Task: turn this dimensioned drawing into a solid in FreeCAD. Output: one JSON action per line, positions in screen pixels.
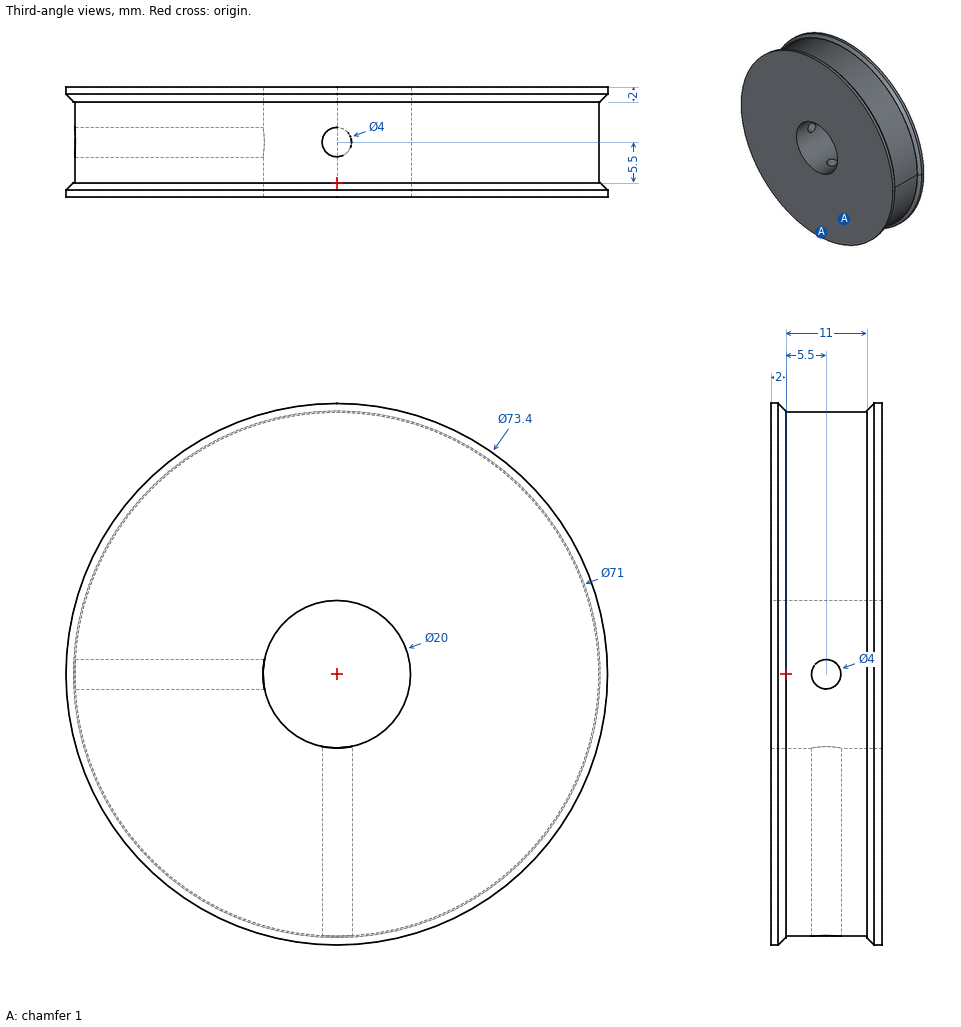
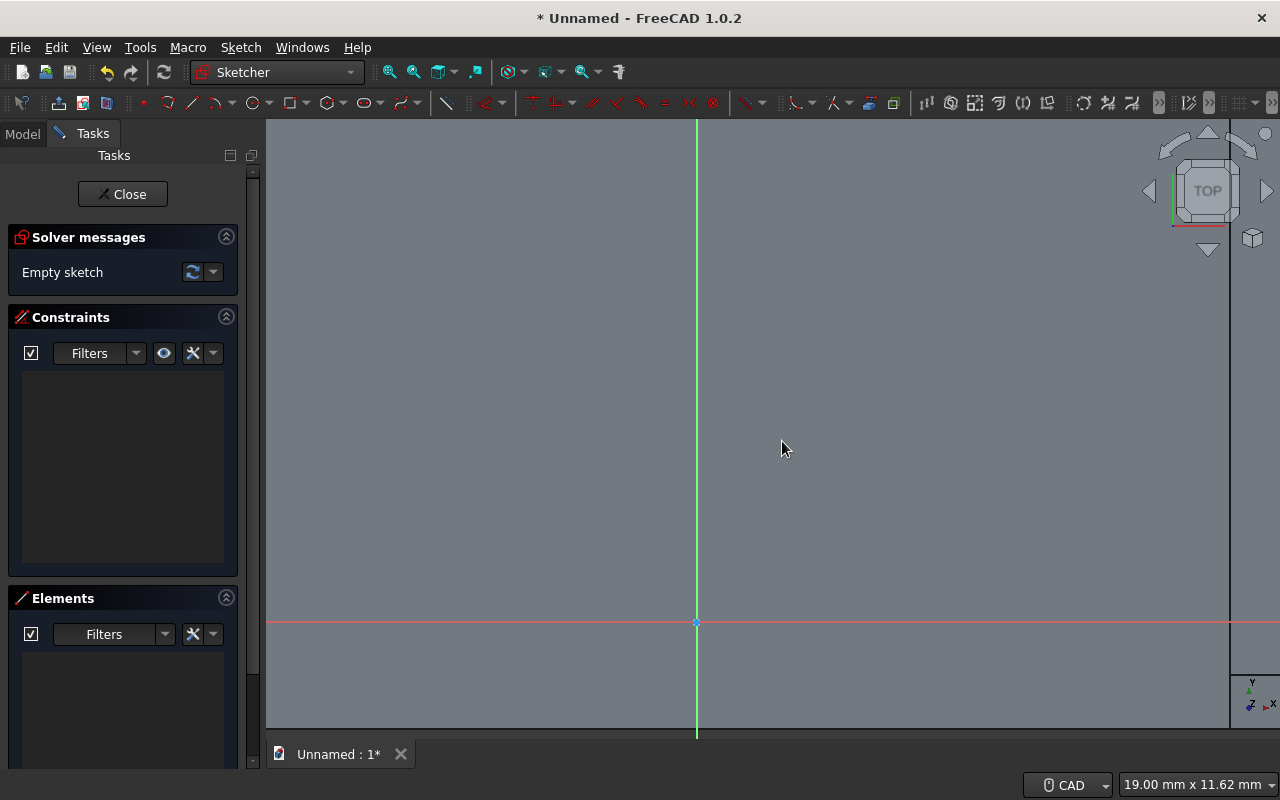
{"action": "left_click", "coordinate": [254, 104]}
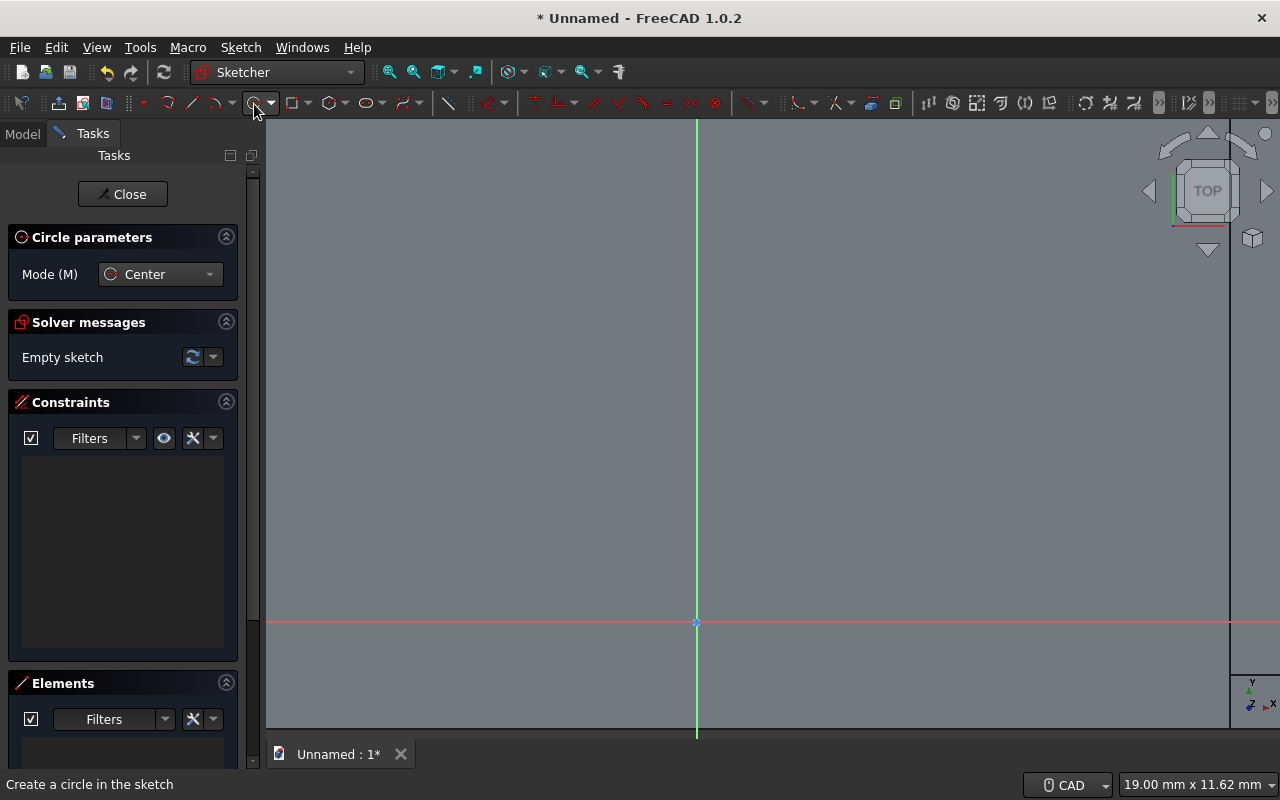
{"action": "left_click", "coordinate": [697, 329]}
{"action": "left_click", "coordinate": [772, 253]}
{"action": "key", "text": "Escape"}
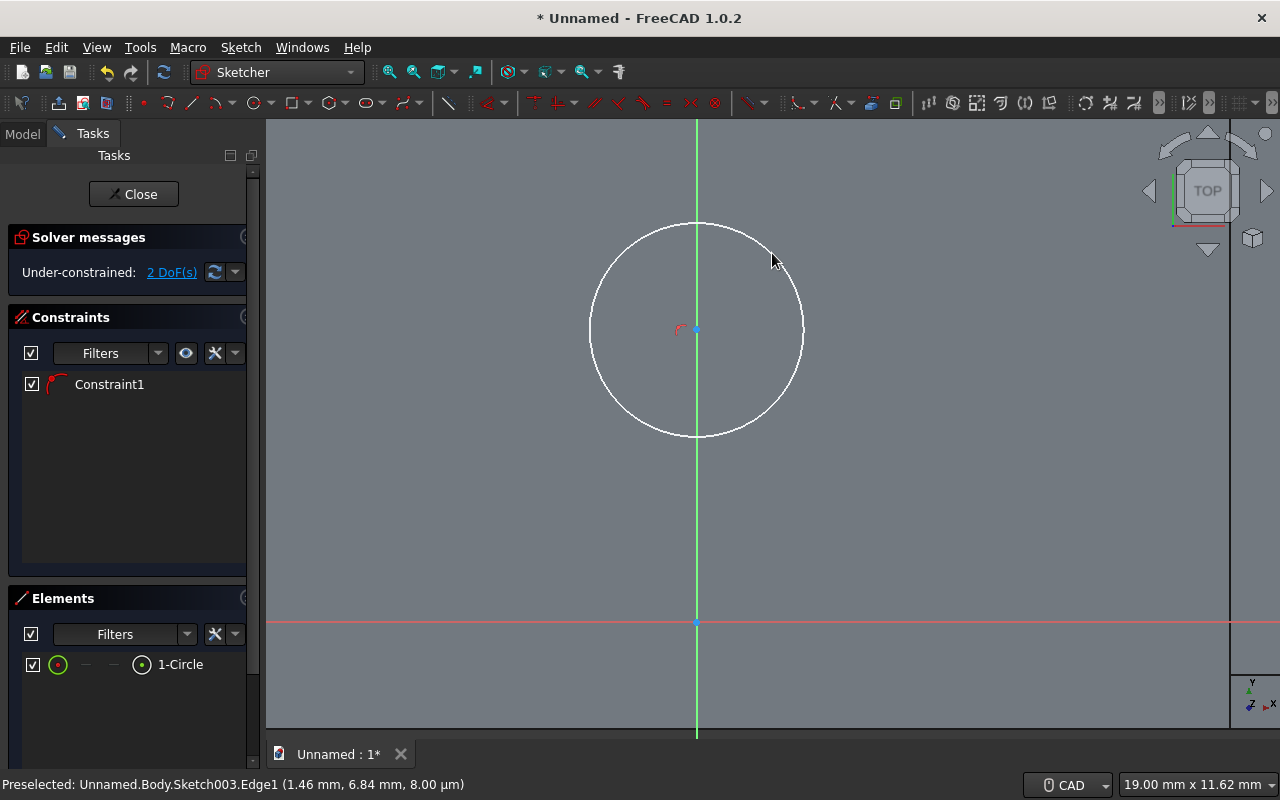
{"action": "left_click", "coordinate": [488, 104]}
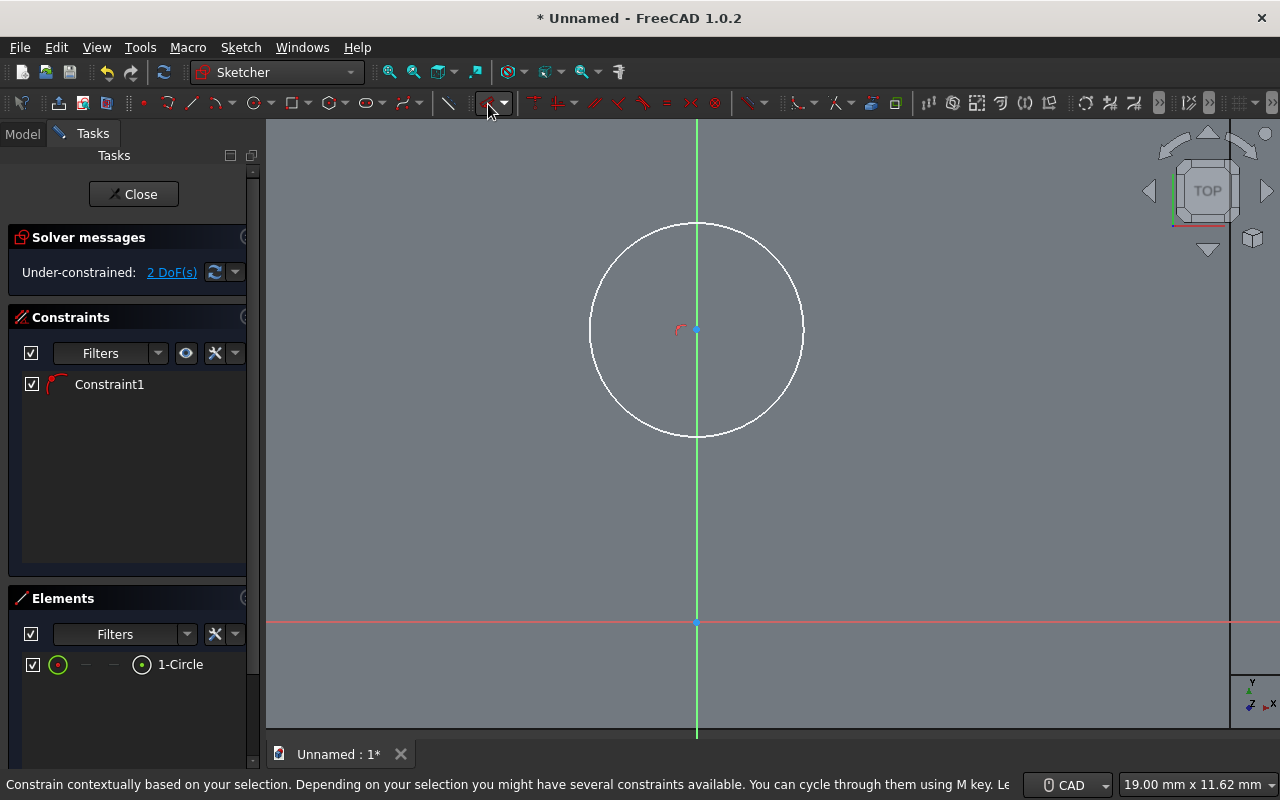
{"action": "left_click", "coordinate": [772, 254]}
{"action": "left_click", "coordinate": [795, 231]}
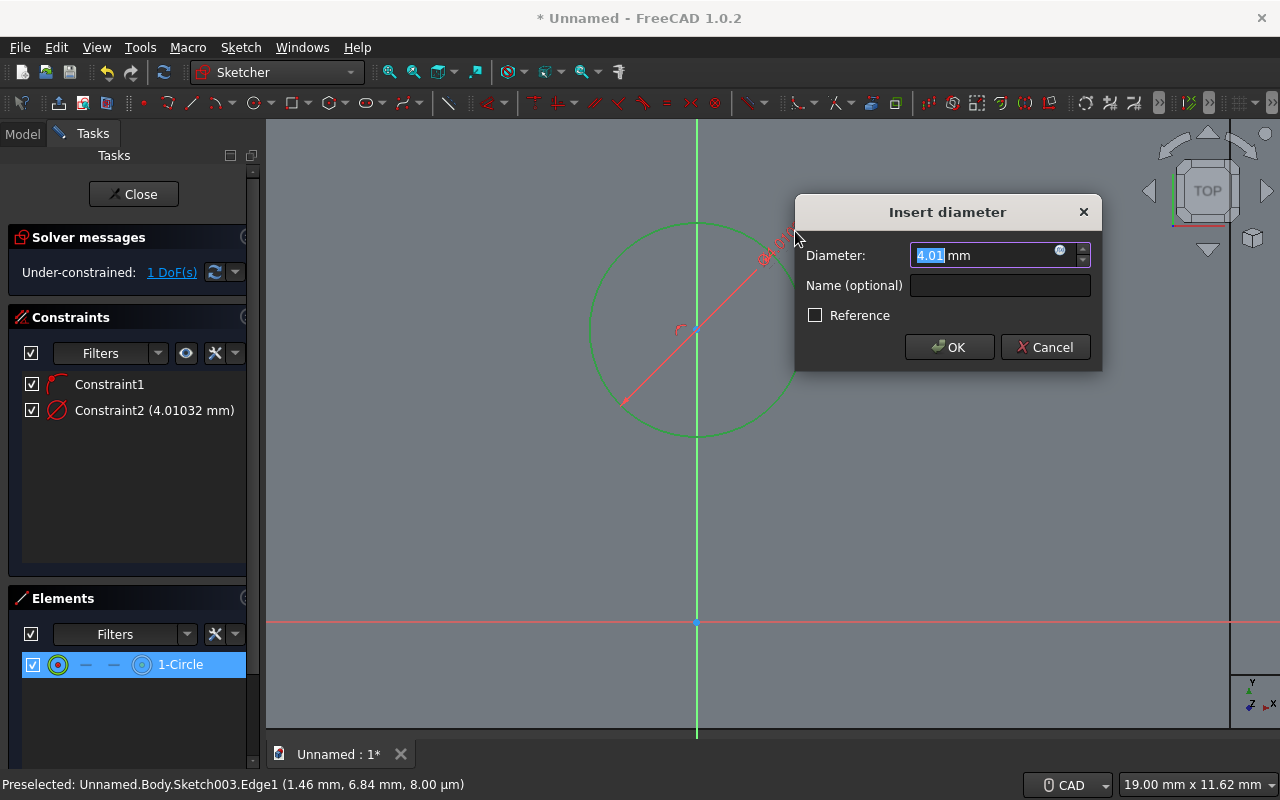
{"action": "type", "text": "4"}
{"action": "key", "text": "Return"}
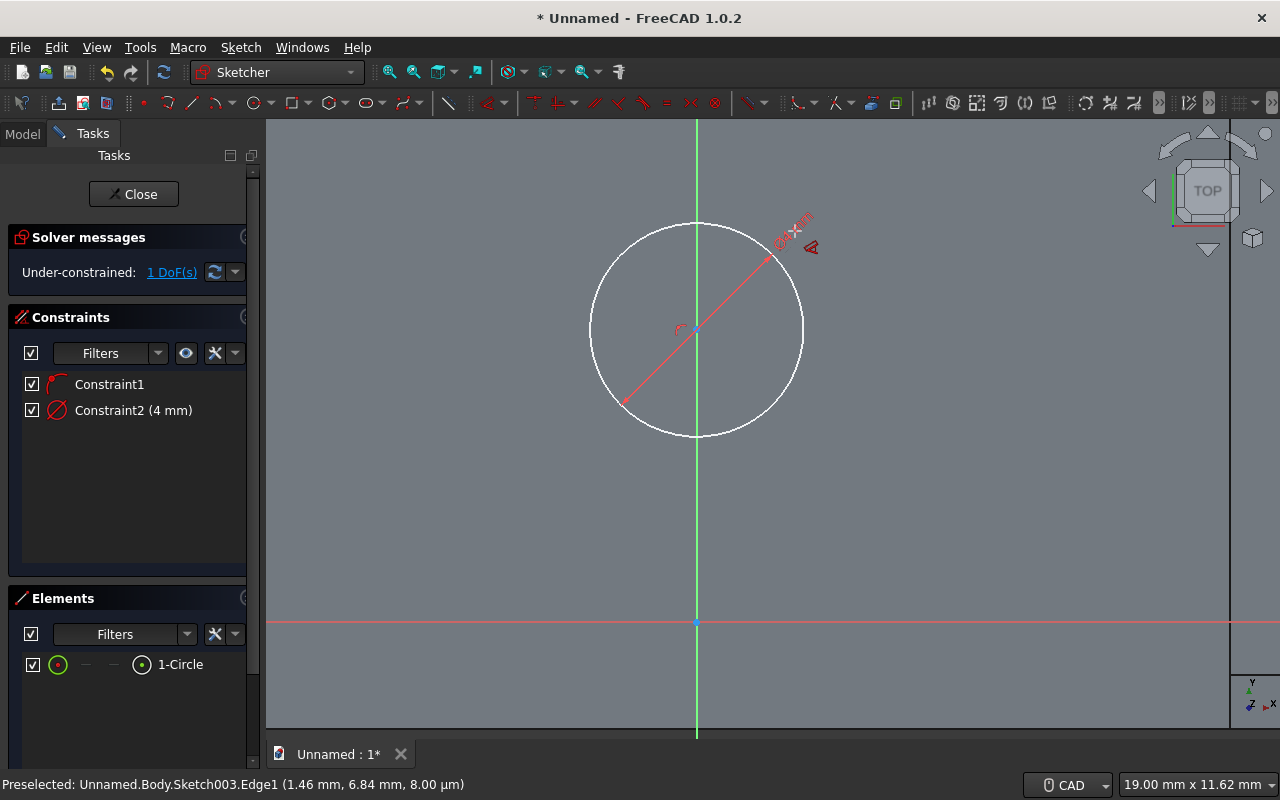
{"action": "left_click", "coordinate": [697, 330]}
{"action": "left_click", "coordinate": [731, 476]}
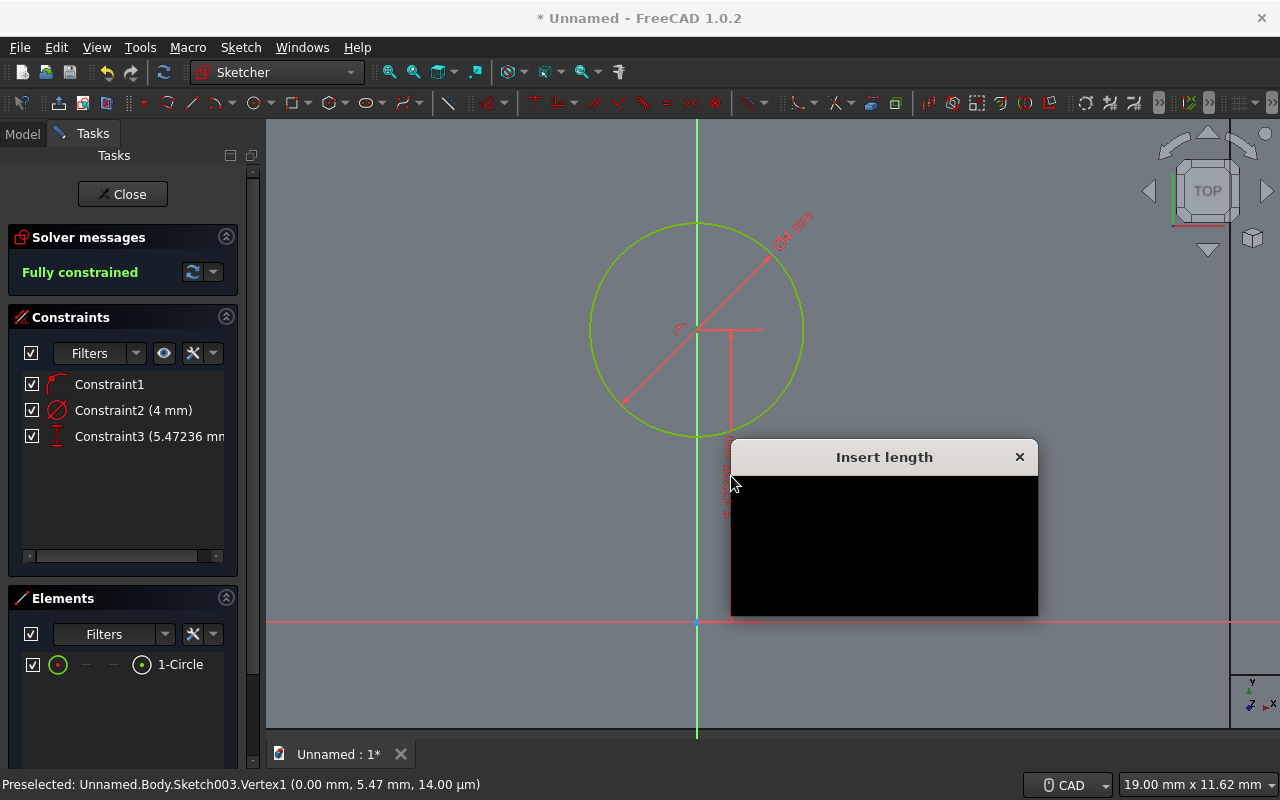
{"action": "type", "text": "5.5"}
{"action": "key", "text": "Return"}
{"action": "key", "text": "Escape"}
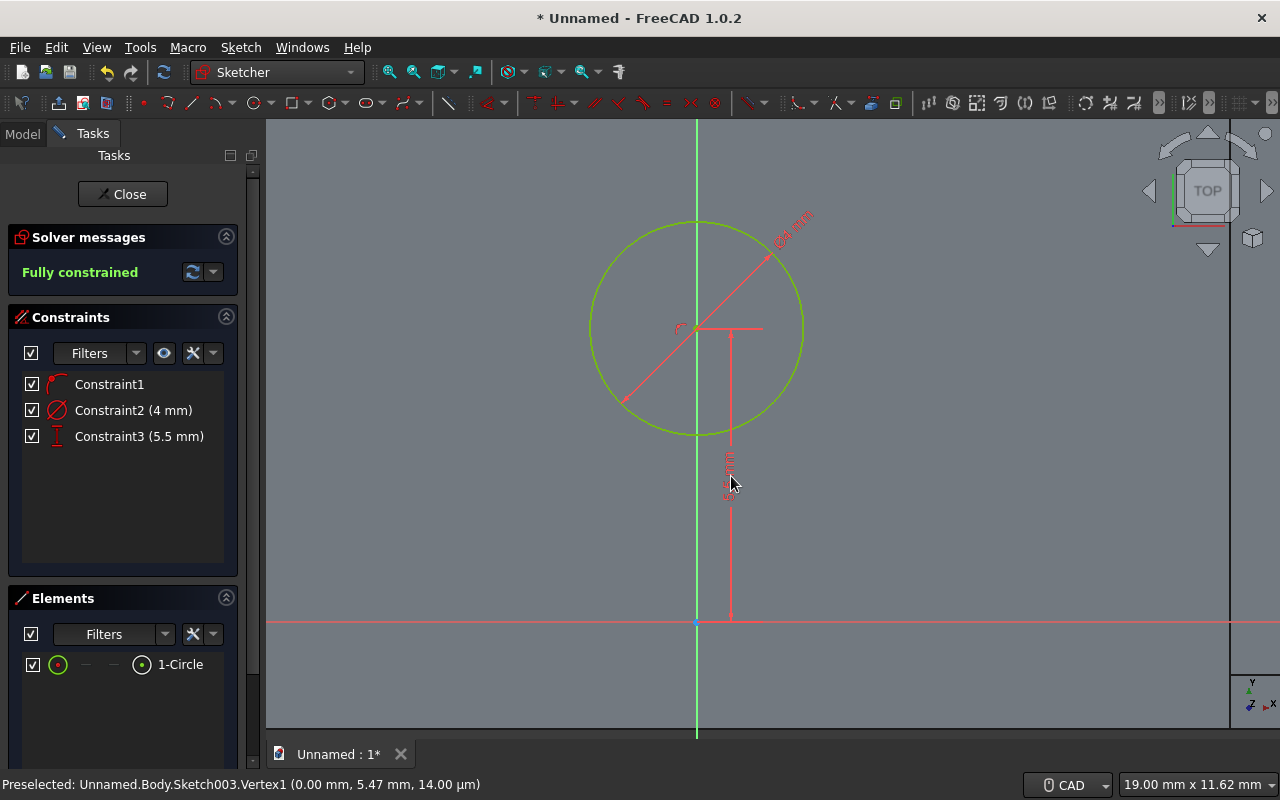
{"action": "left_click", "coordinate": [123, 194]}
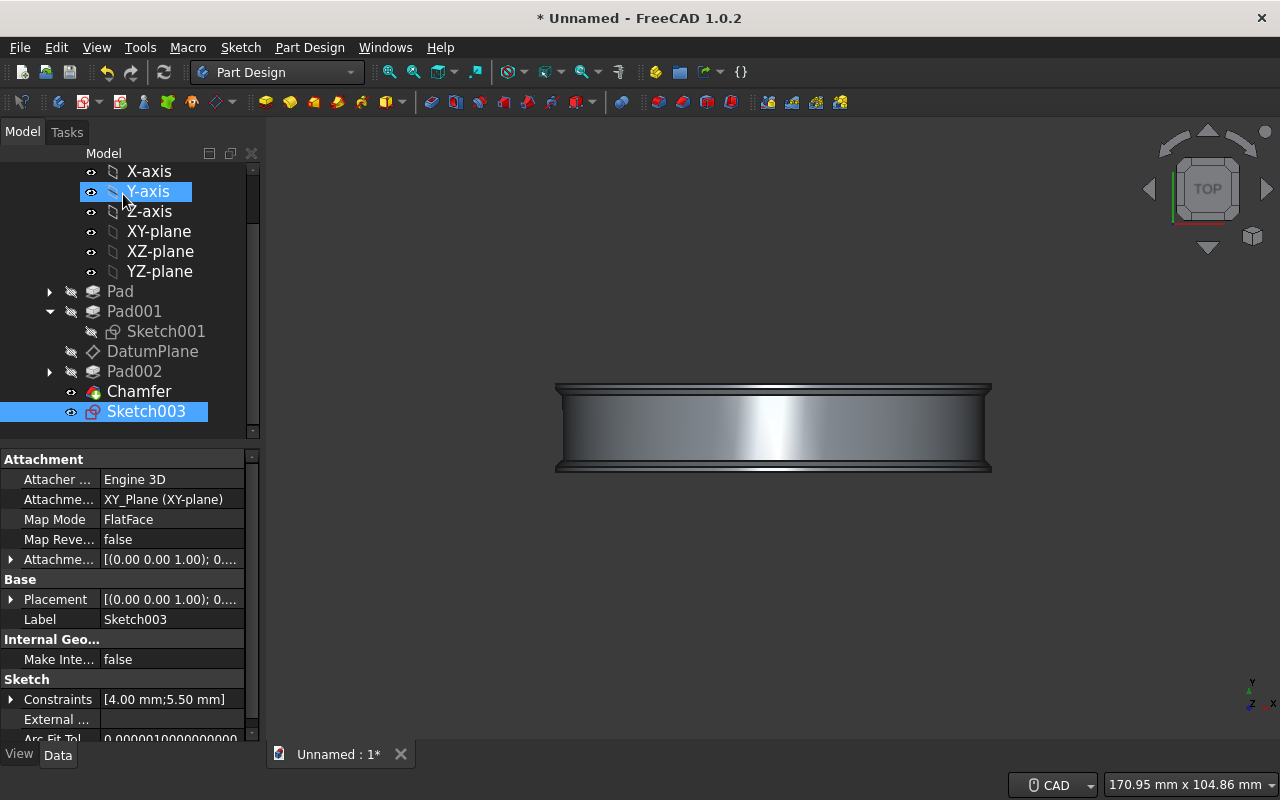
{"action": "left_click", "coordinate": [432, 102]}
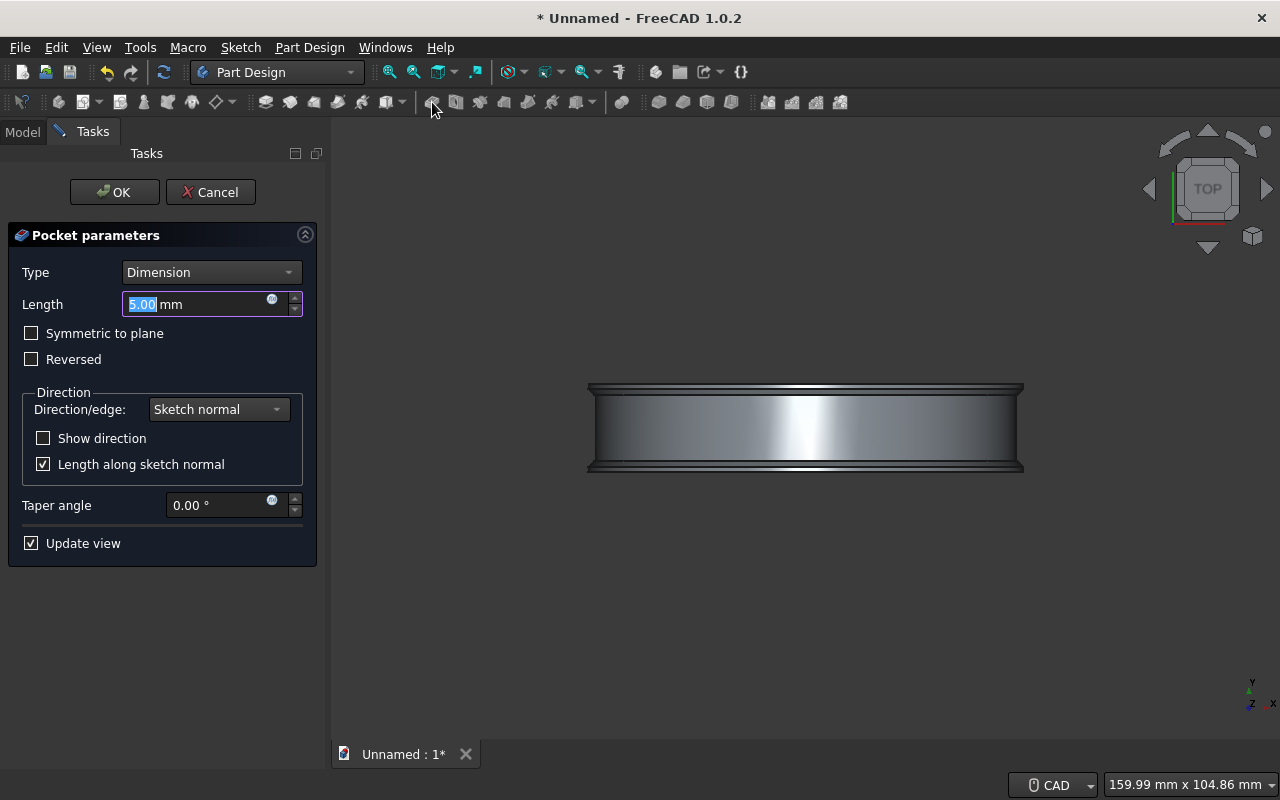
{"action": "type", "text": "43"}
{"action": "key", "text": "Tab"}